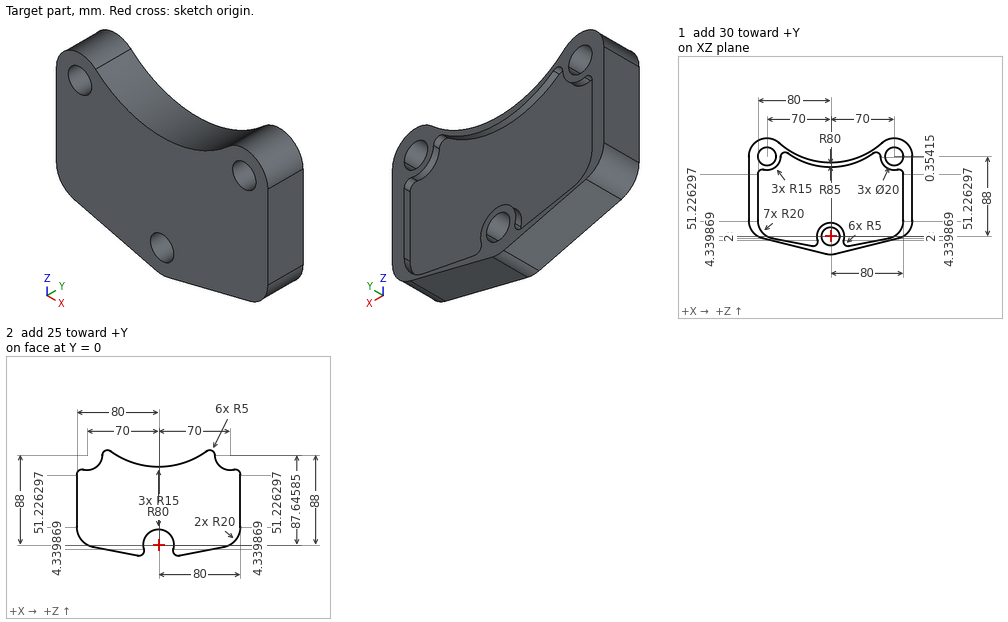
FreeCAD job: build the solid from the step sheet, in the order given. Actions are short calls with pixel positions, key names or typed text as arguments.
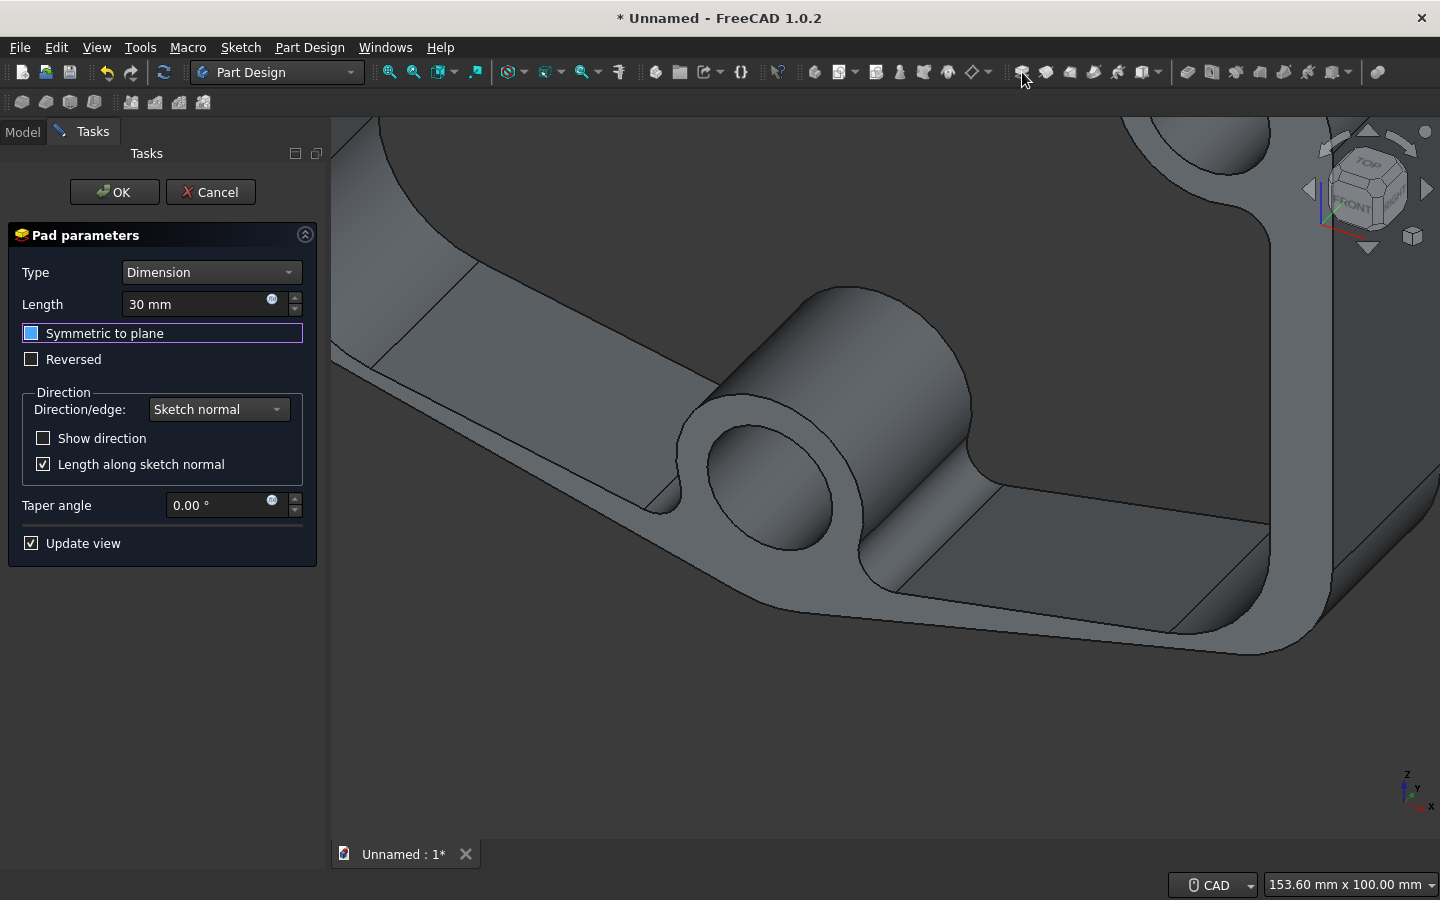
click(30, 359)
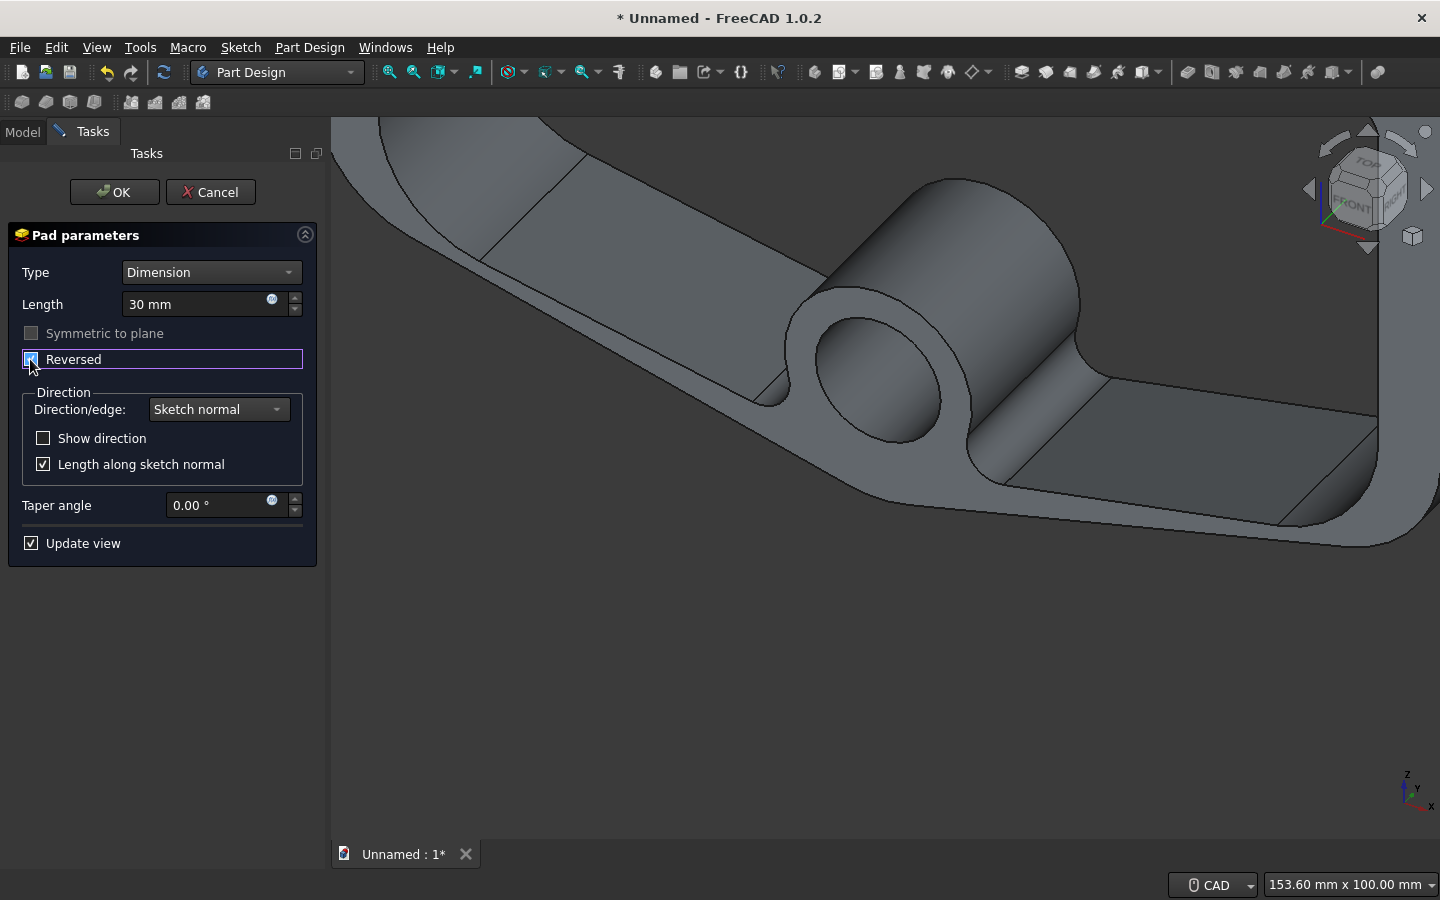
click(115, 192)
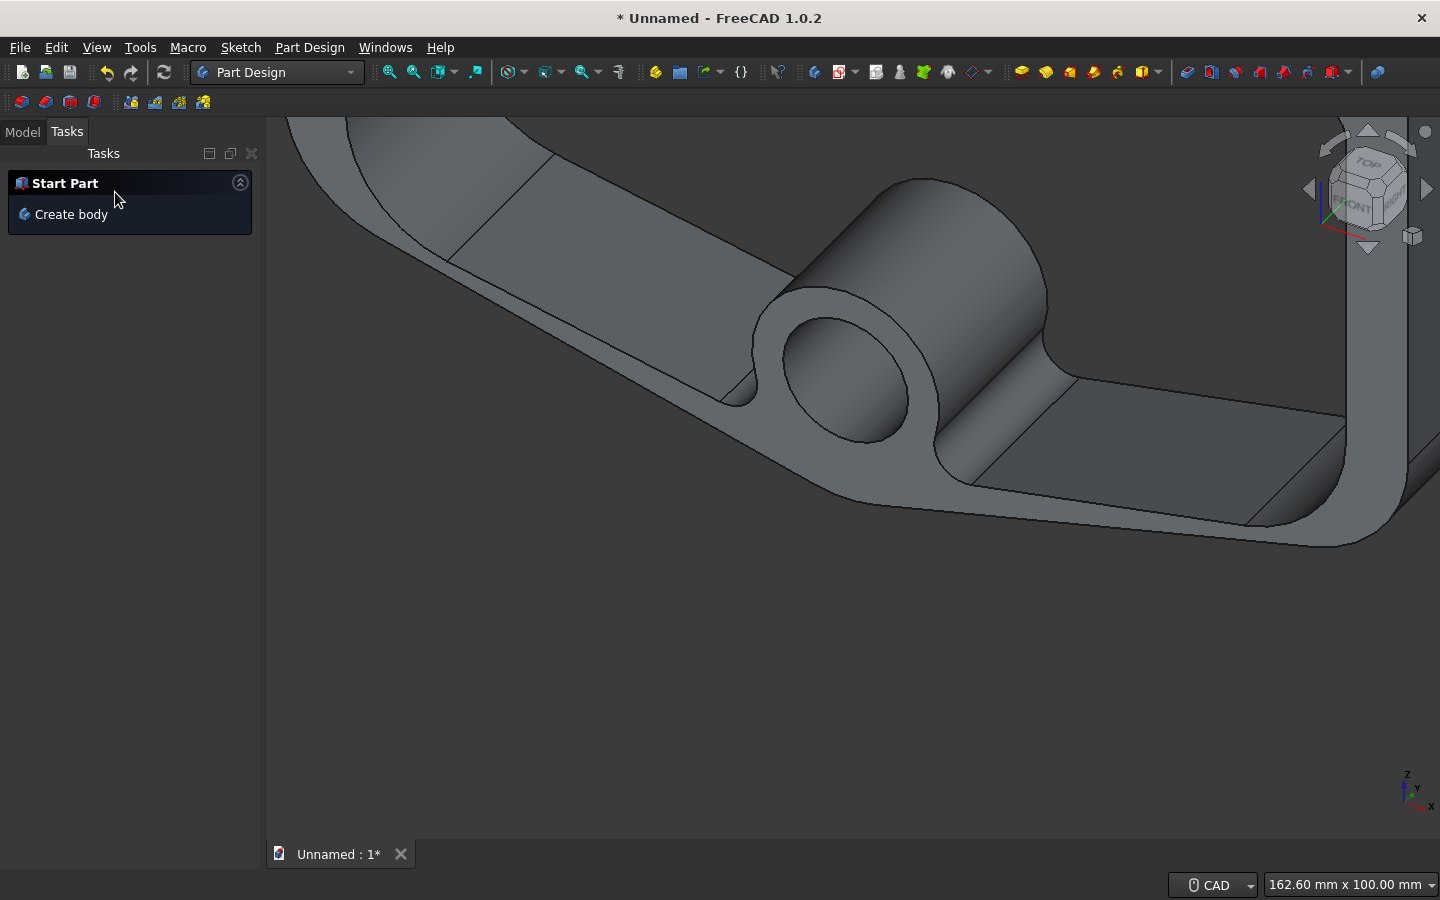
click(390, 72)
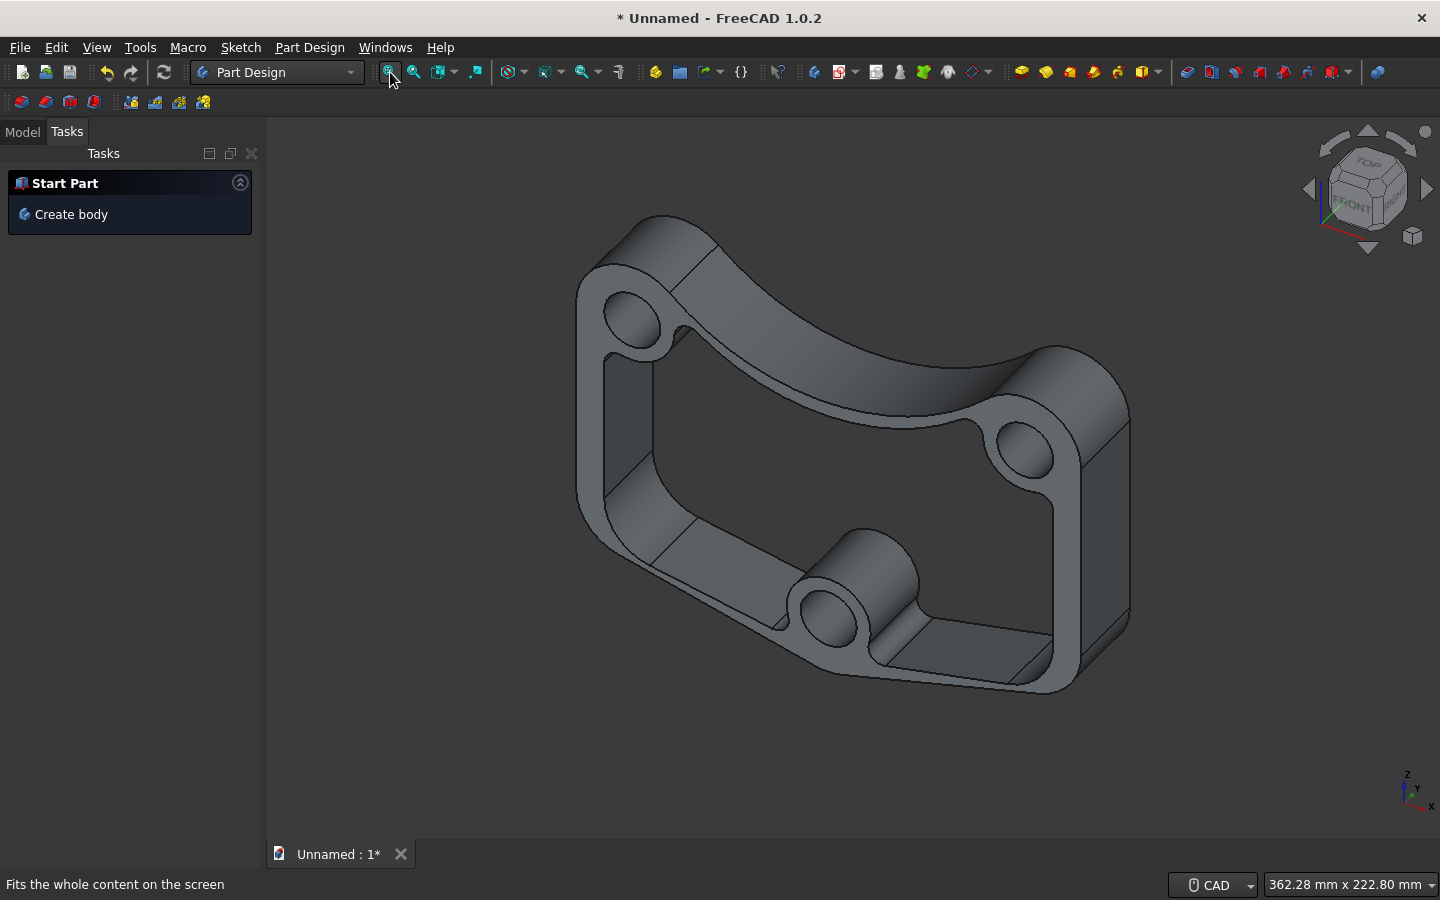
click(1045, 427)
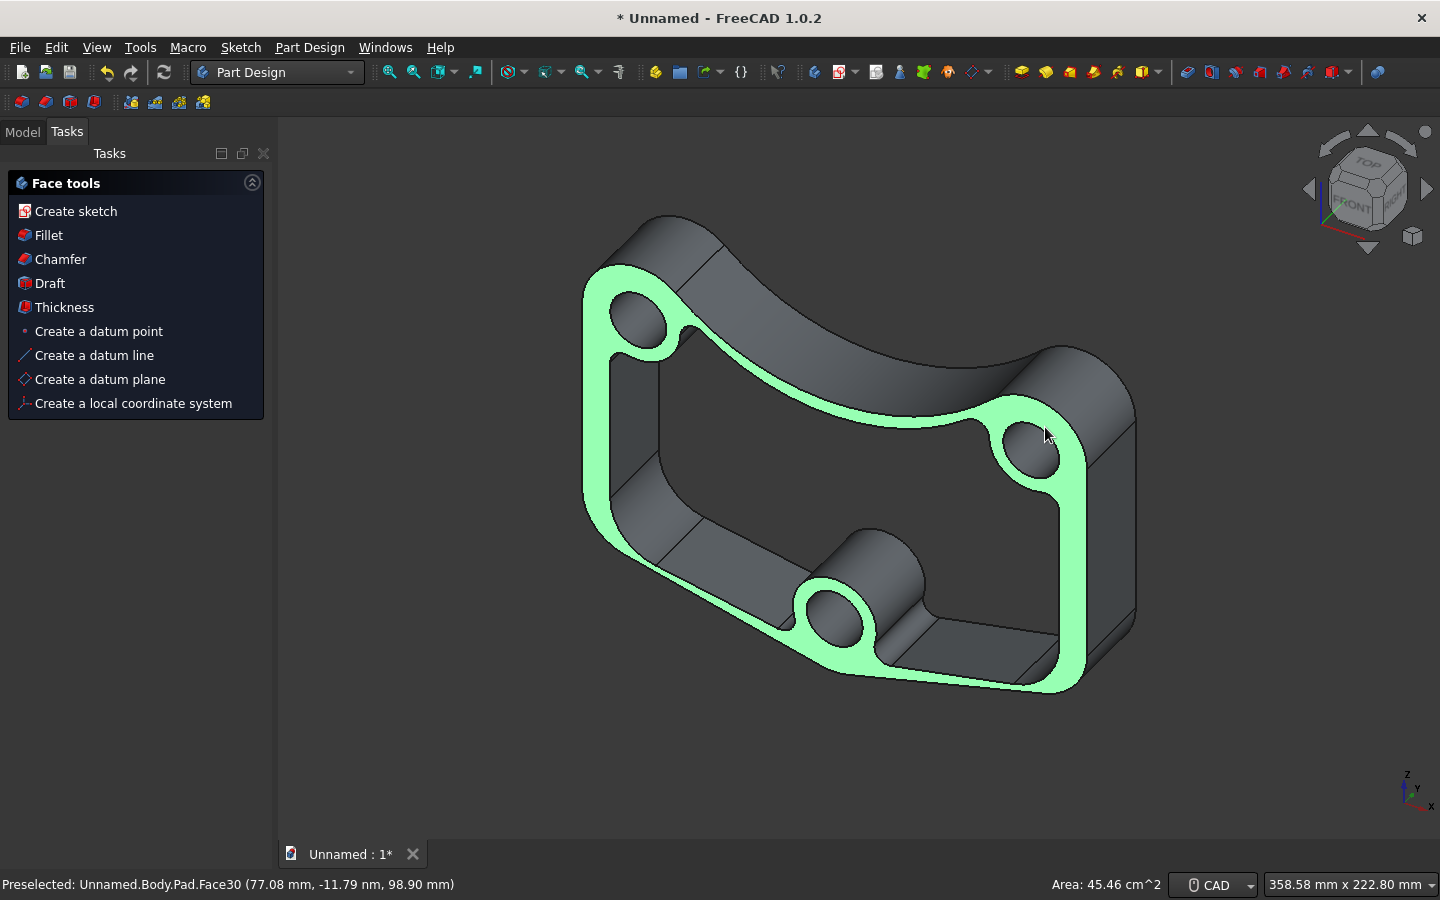
click(840, 72)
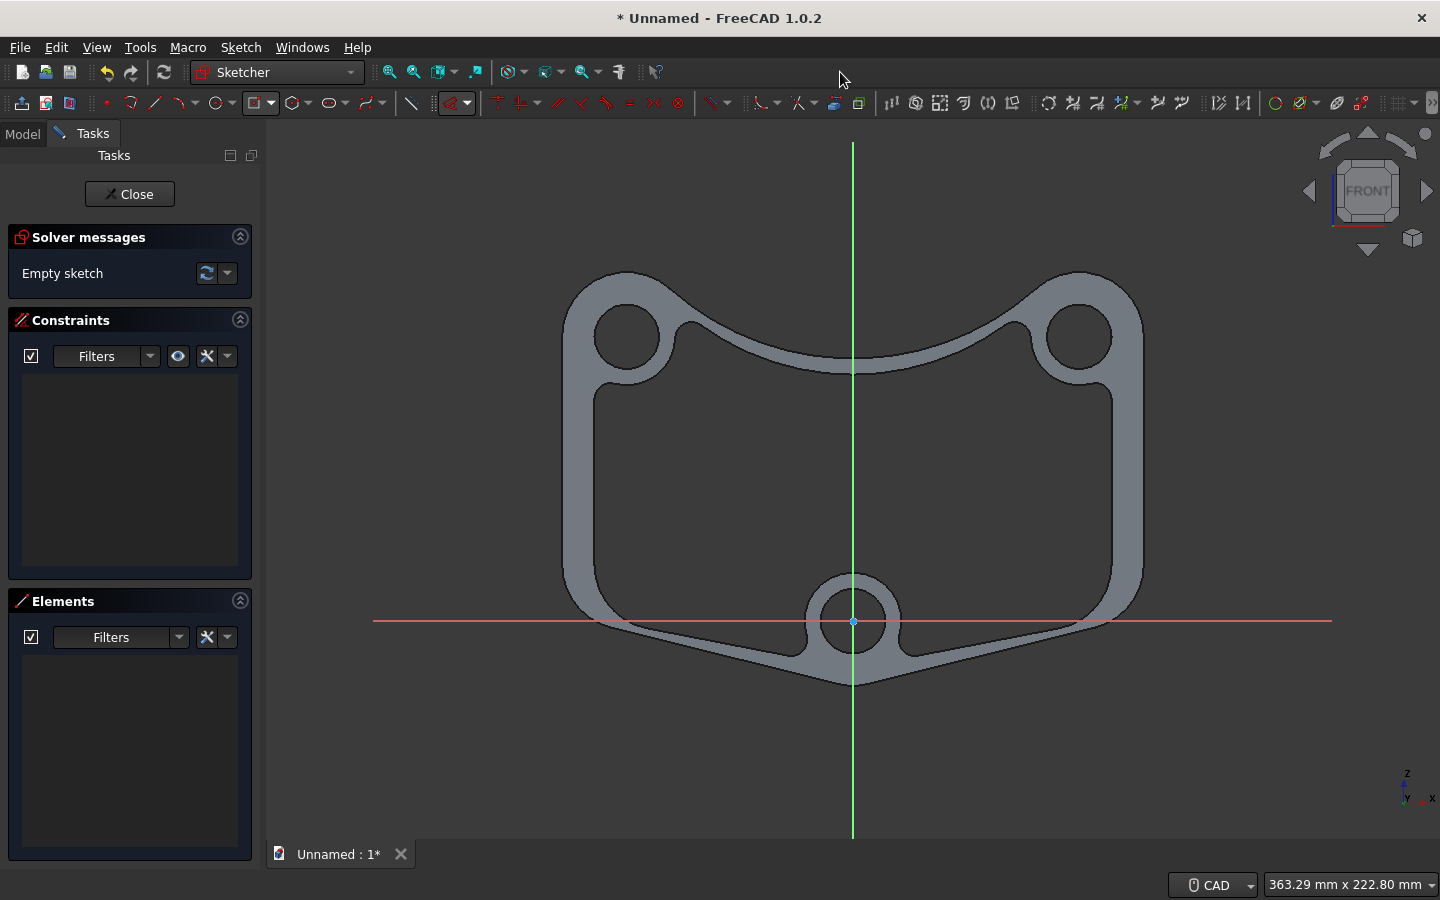
click(156, 104)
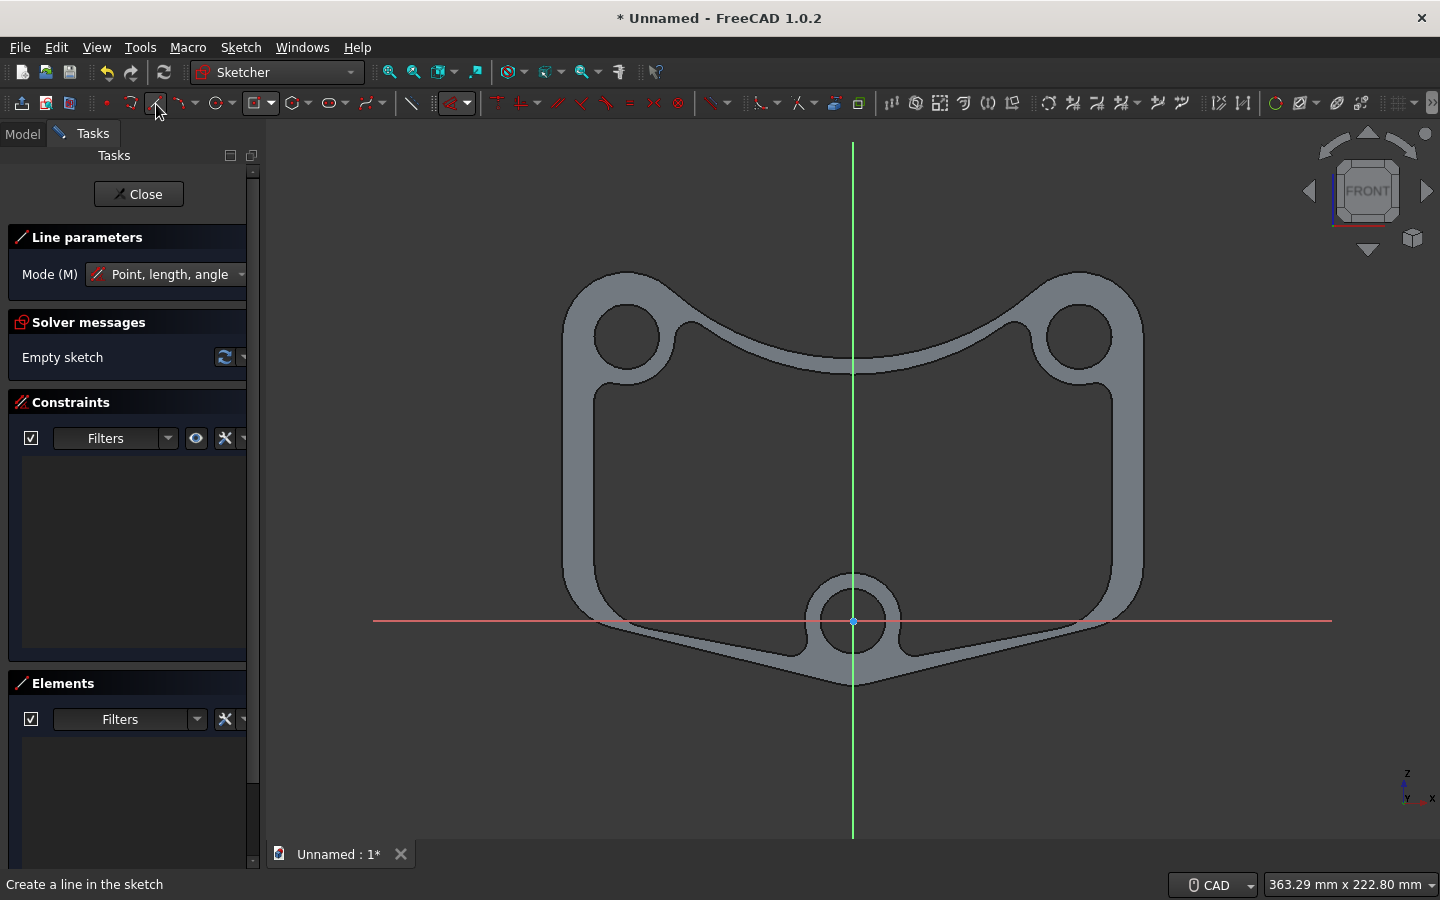
scroll(647, 628, up, 4)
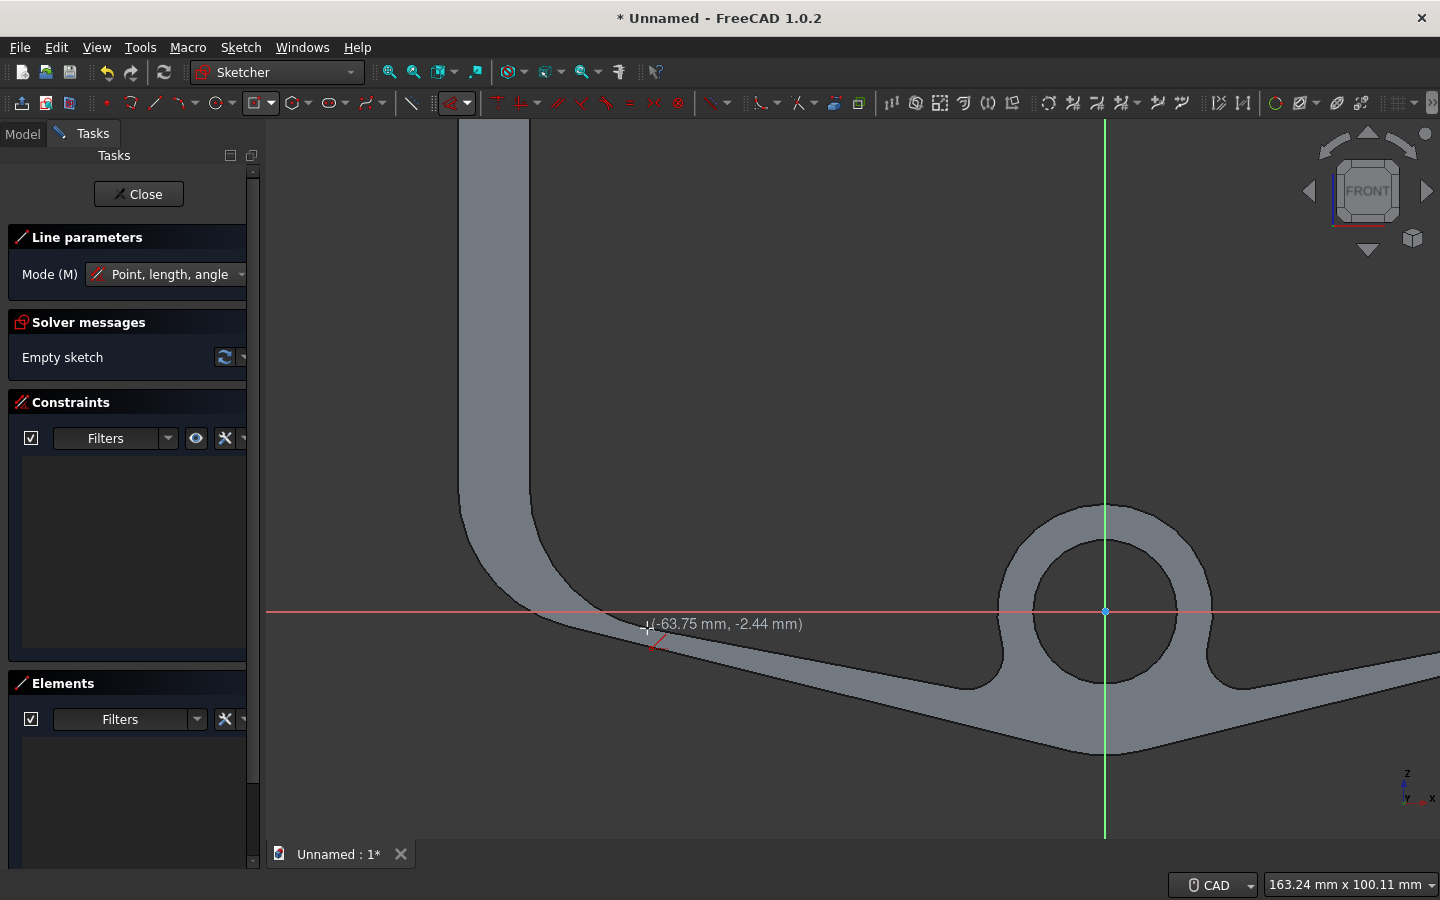
click(646, 628)
click(961, 689)